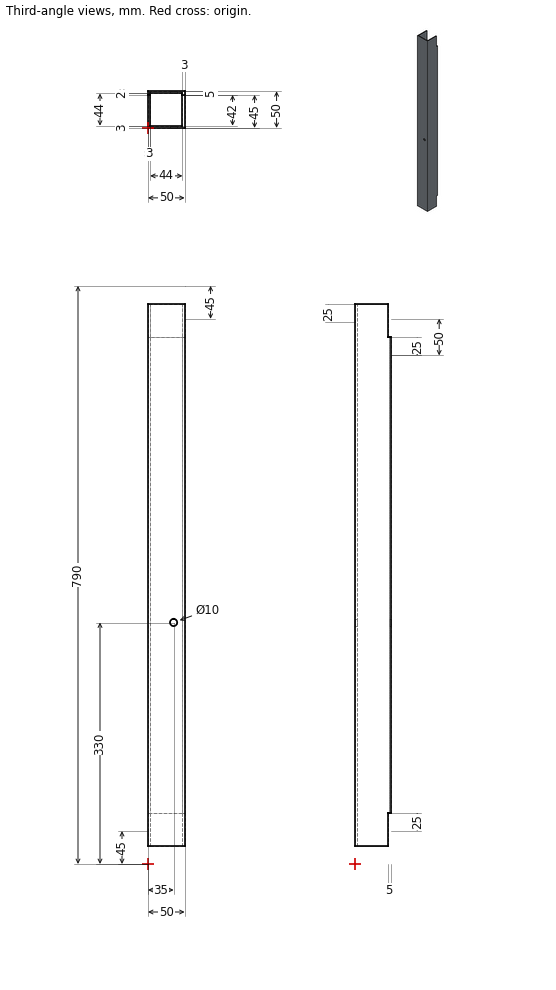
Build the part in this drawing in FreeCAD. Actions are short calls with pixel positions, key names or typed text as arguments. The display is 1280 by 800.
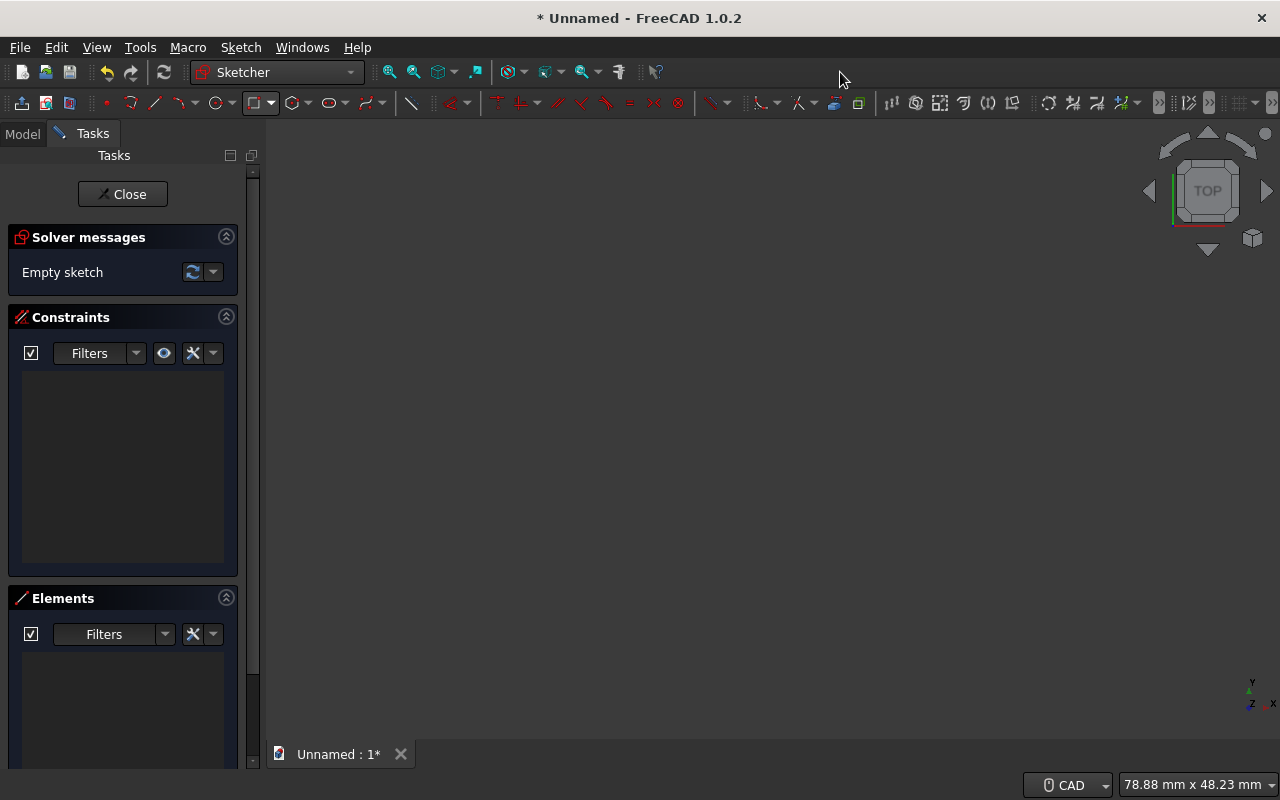
scroll(704, 429, down, 5)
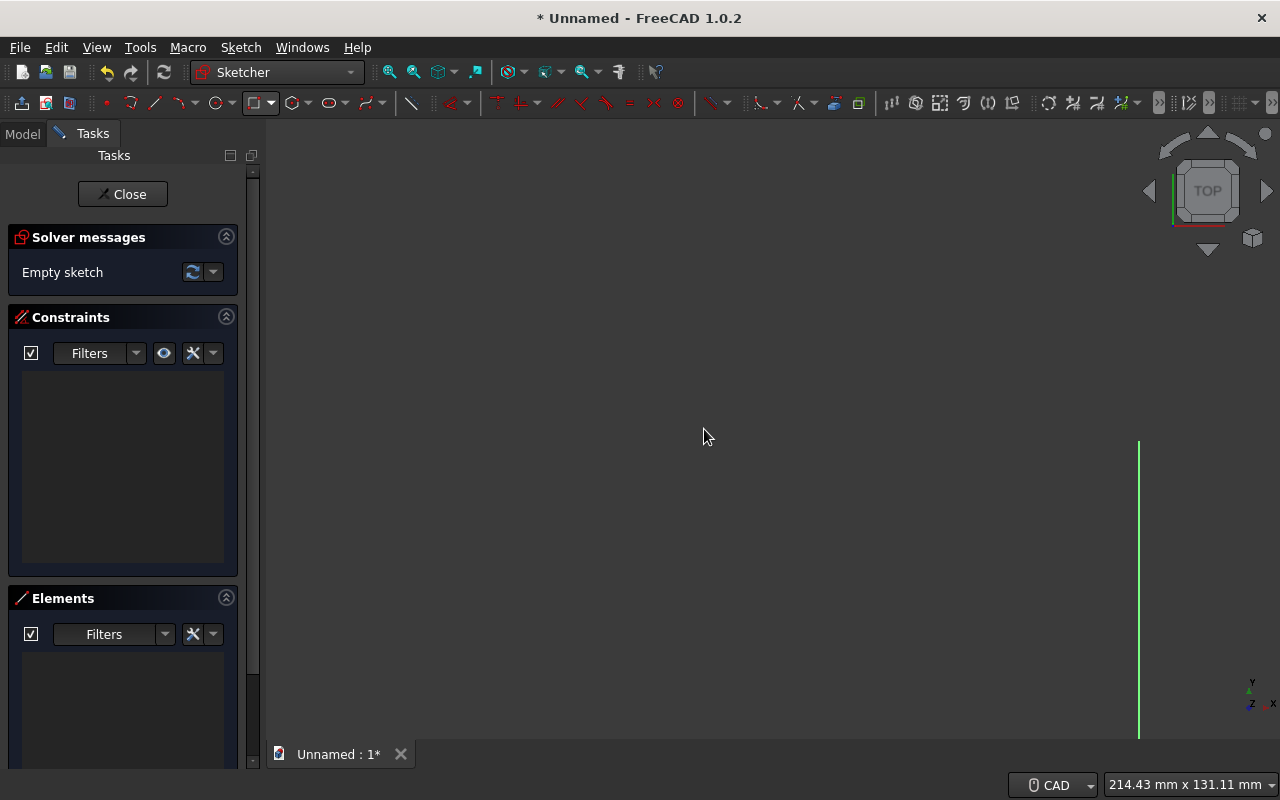
scroll(704, 429, down, 5)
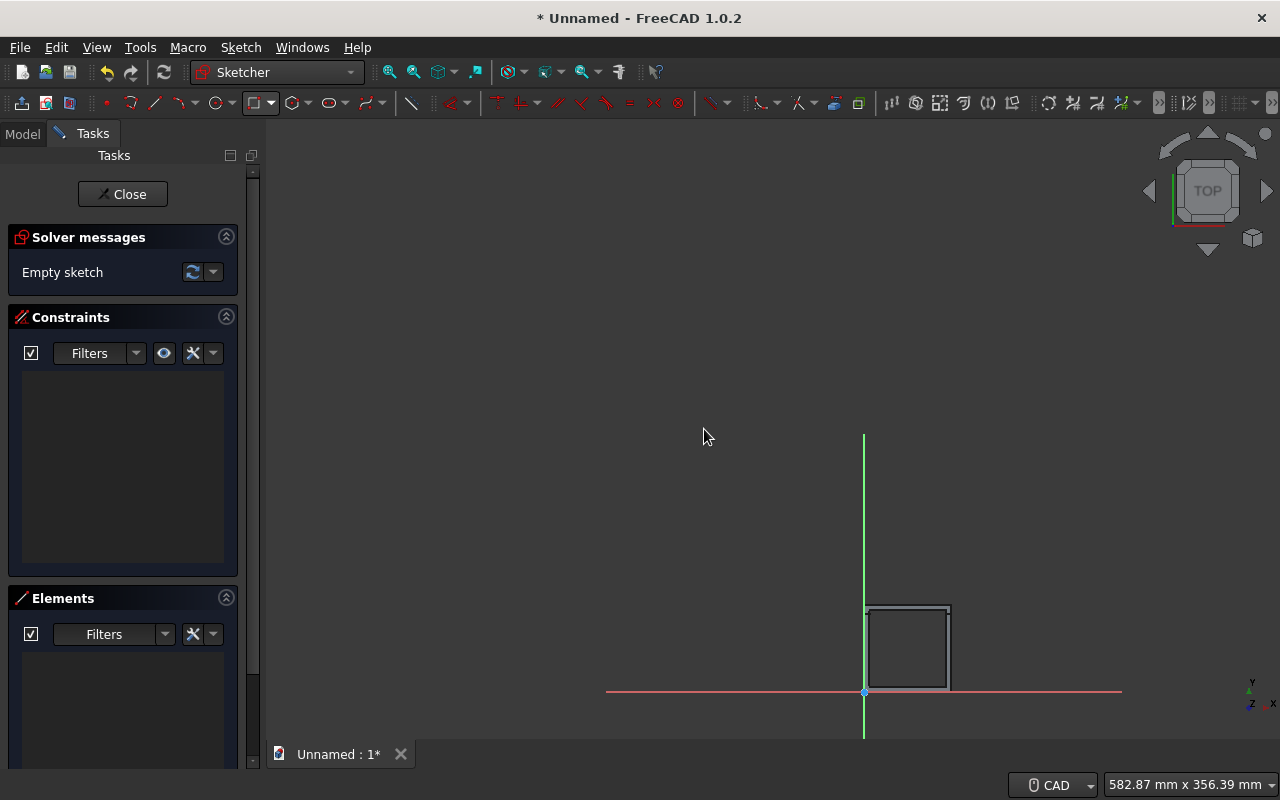
scroll(959, 710, up, 8)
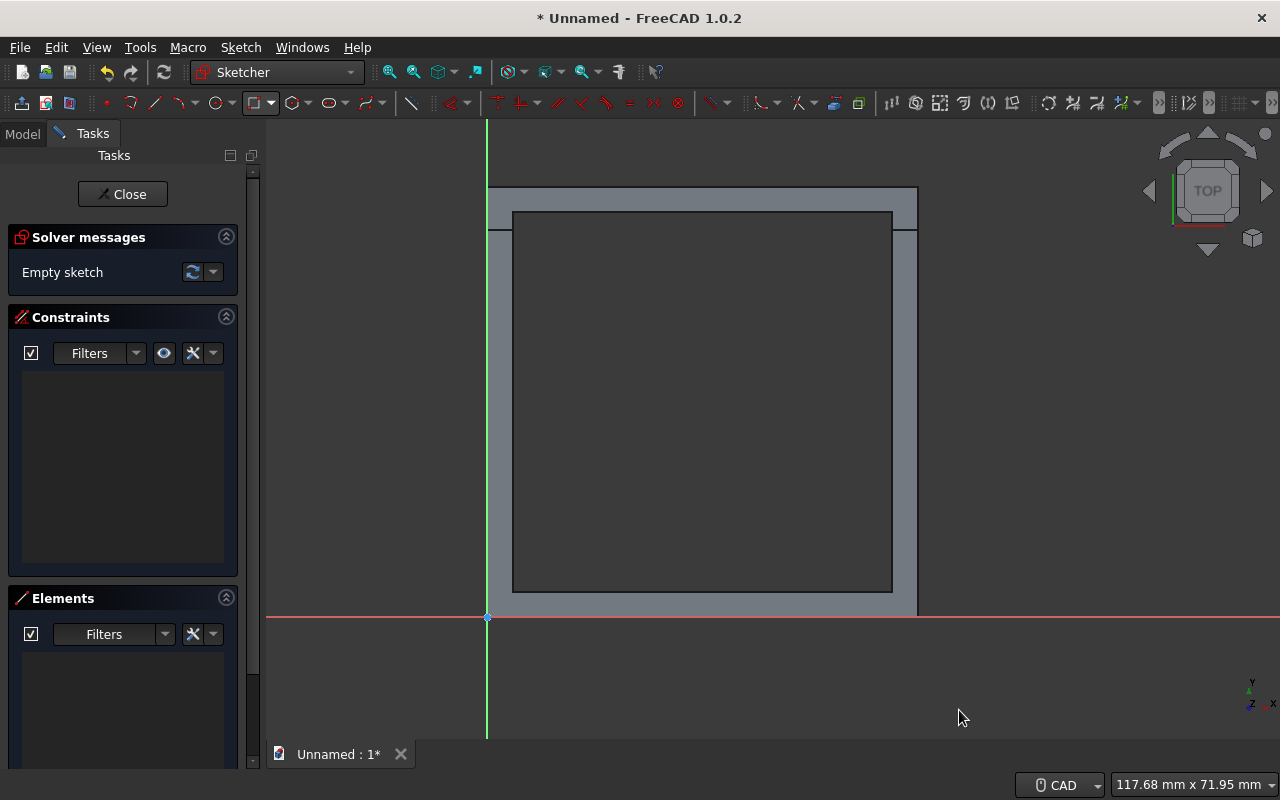
click(132, 104)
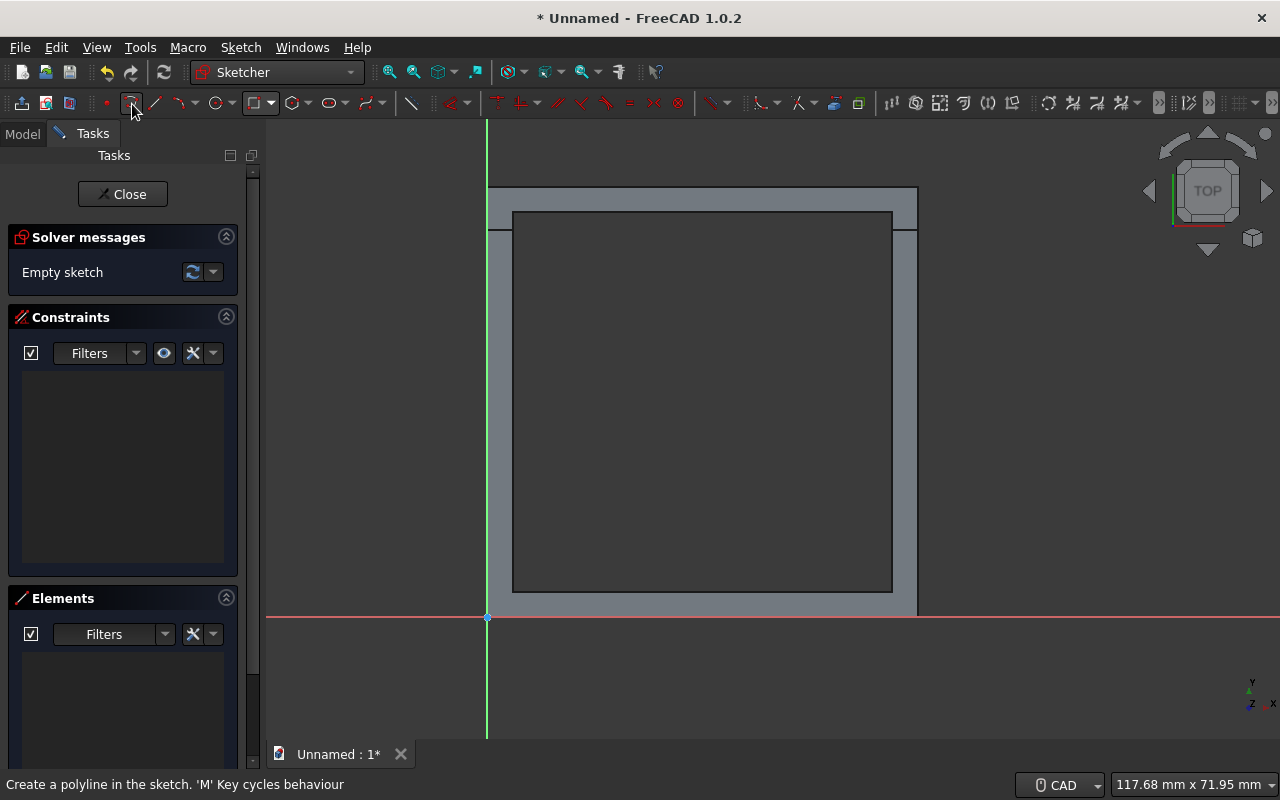
click(487, 617)
click(918, 608)
click(918, 230)
click(892, 230)
click(892, 592)
click(513, 592)
click(513, 230)
click(496, 230)
click(487, 617)
key(Escape)
key(Escape)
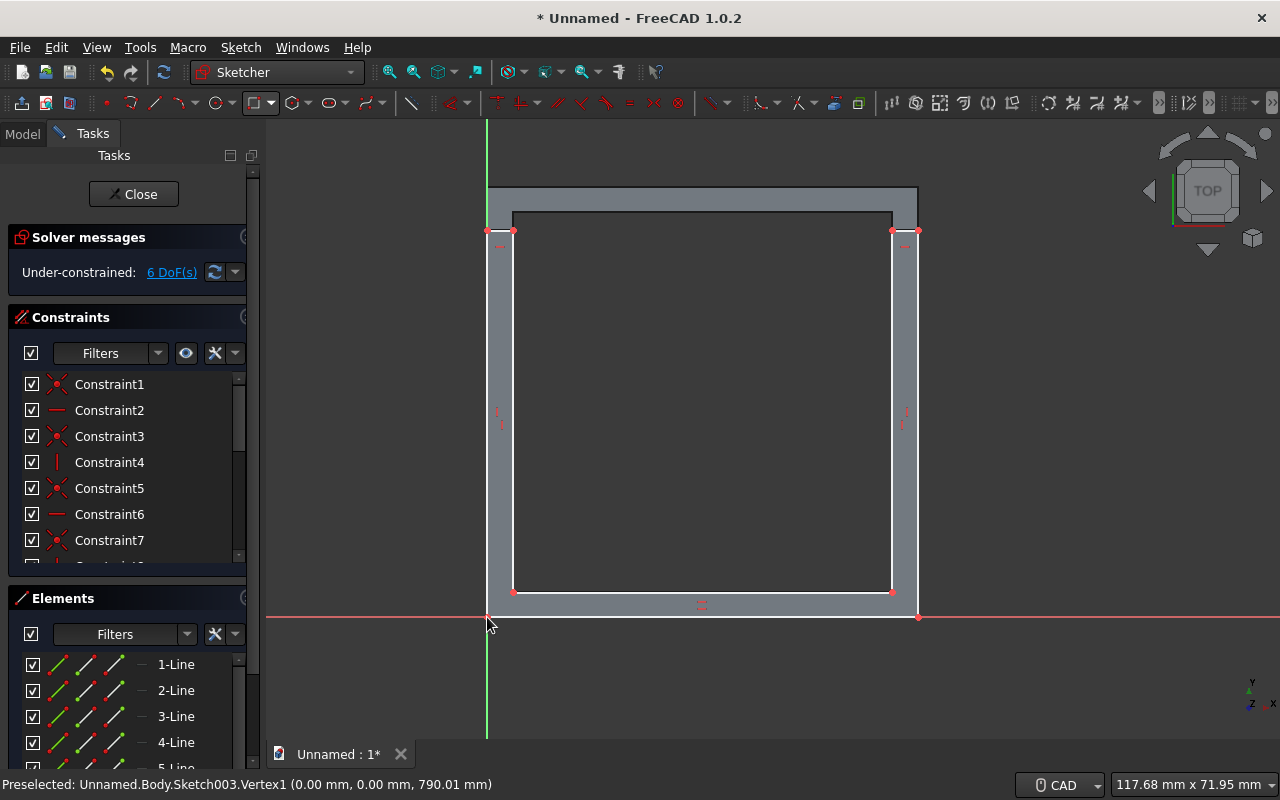
click(450, 104)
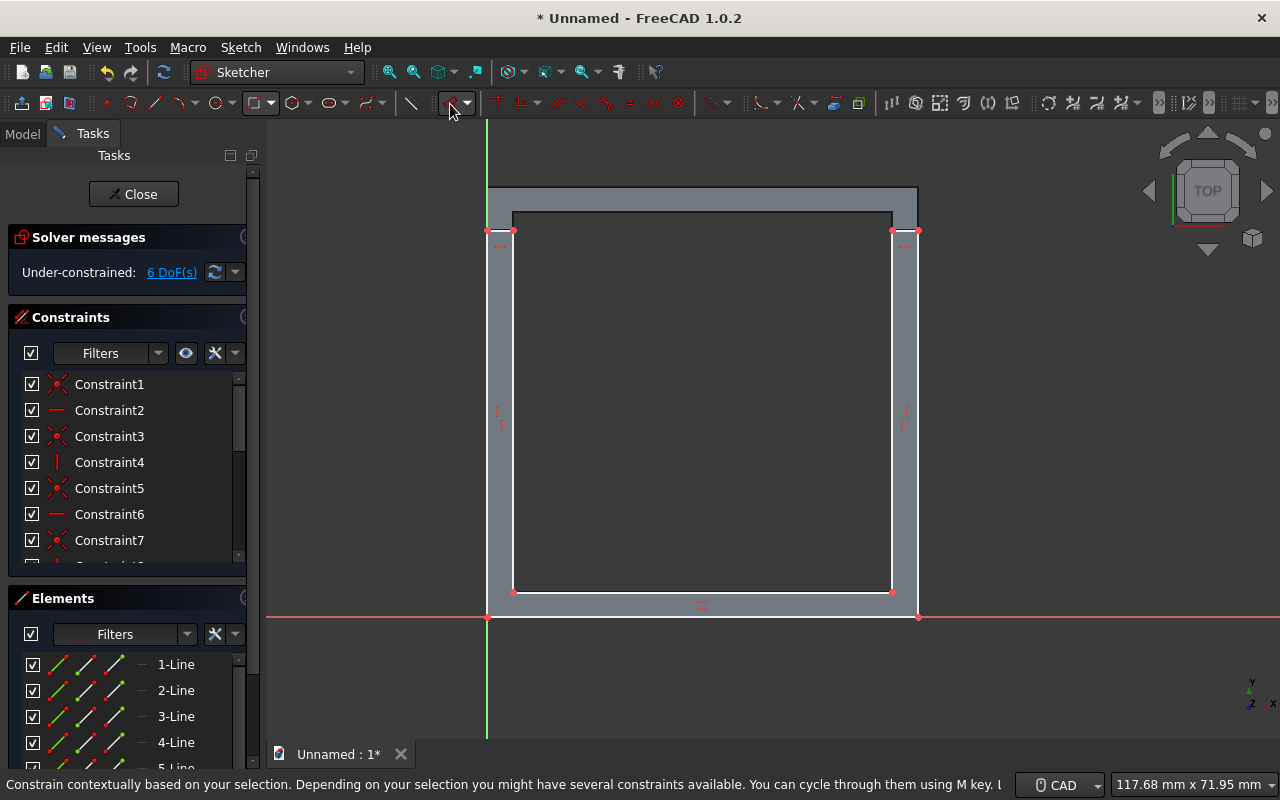
scroll(908, 231, up, 3)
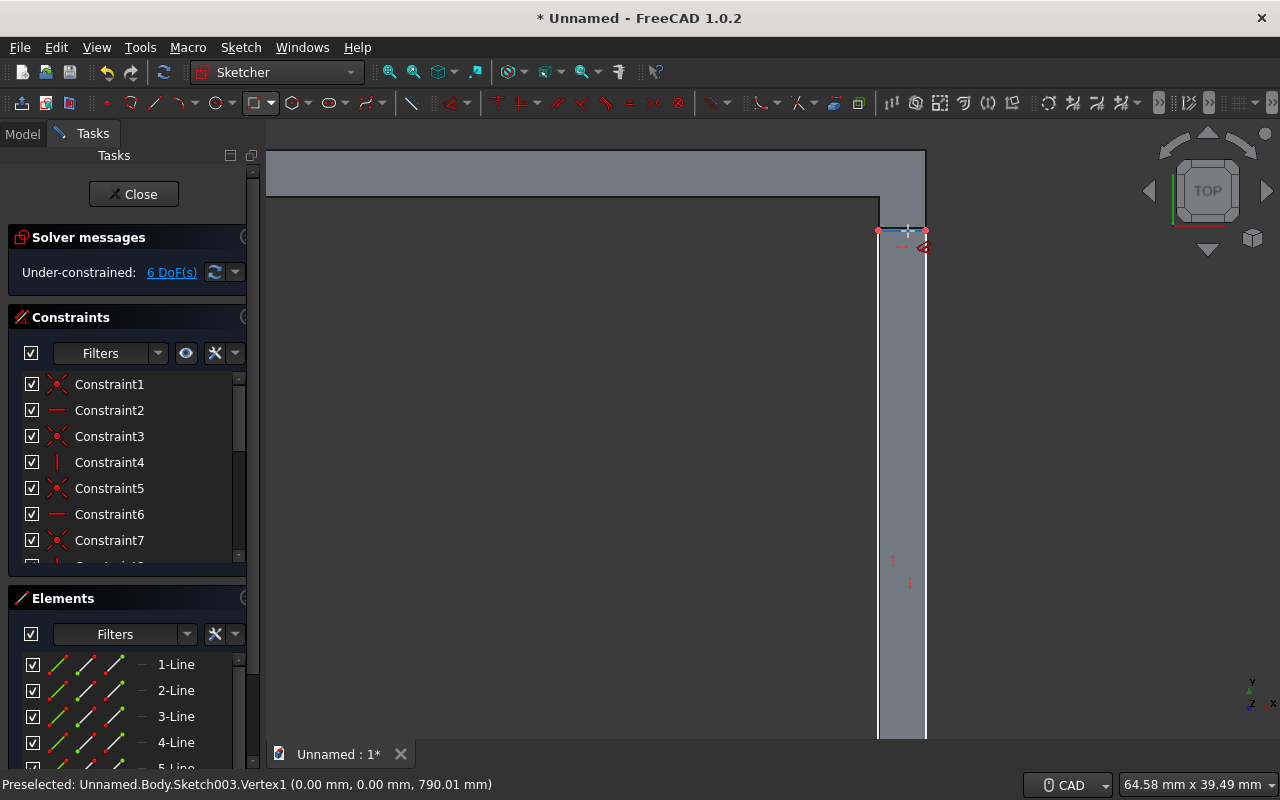
click(907, 231)
click(902, 197)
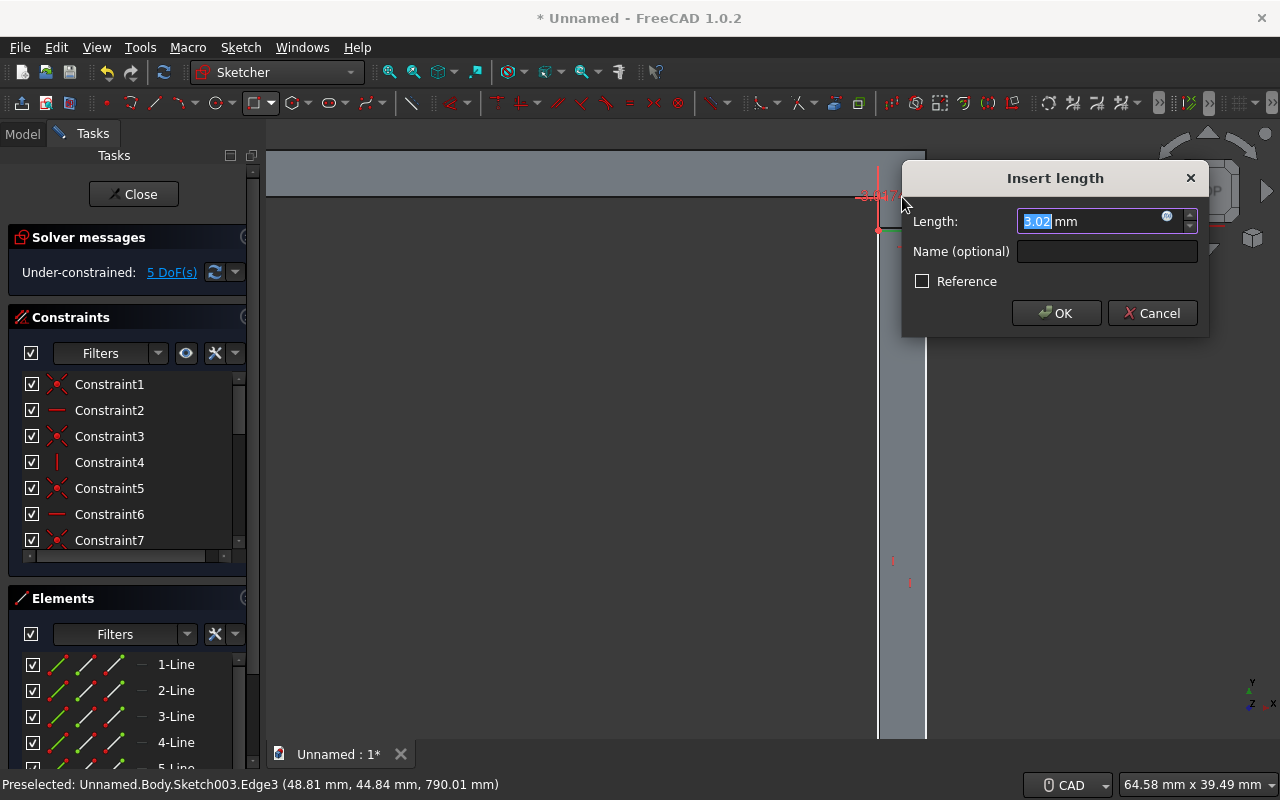
text(3)
key(Return)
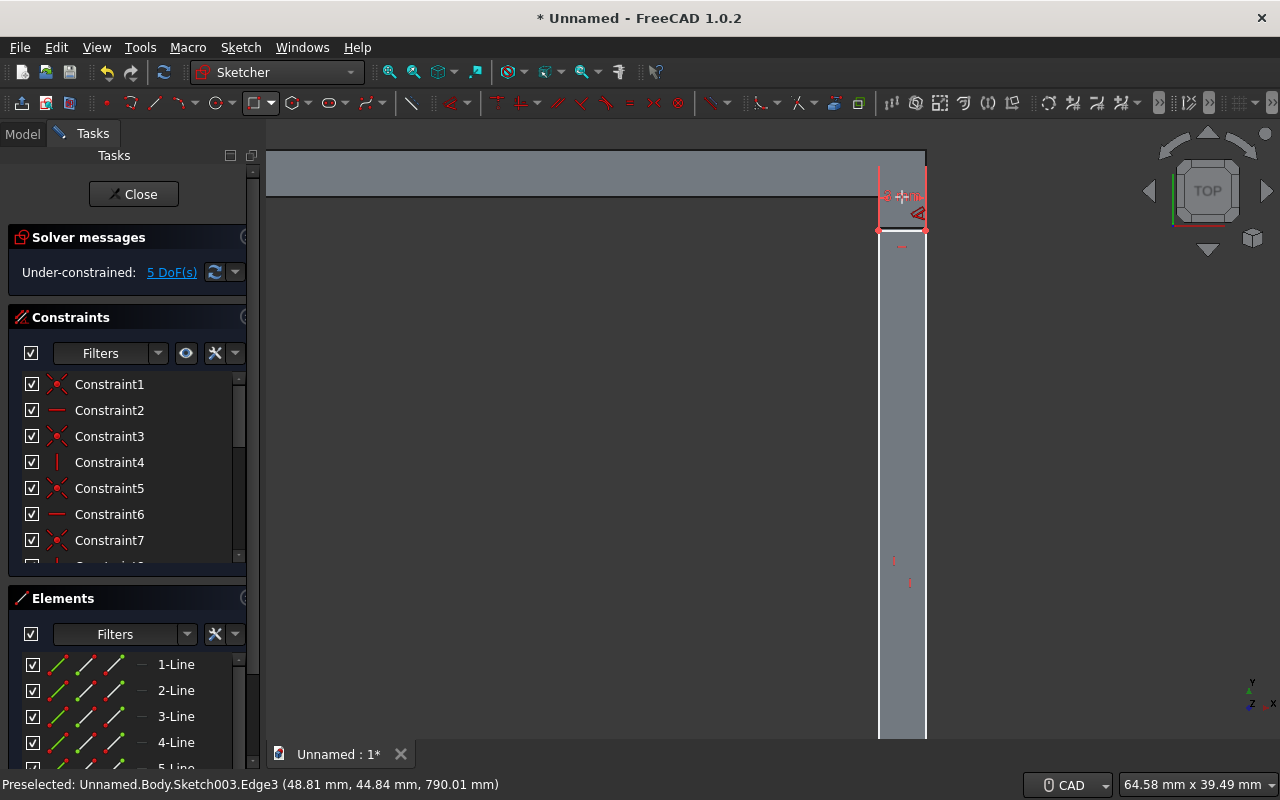
scroll(913, 243, down, 3)